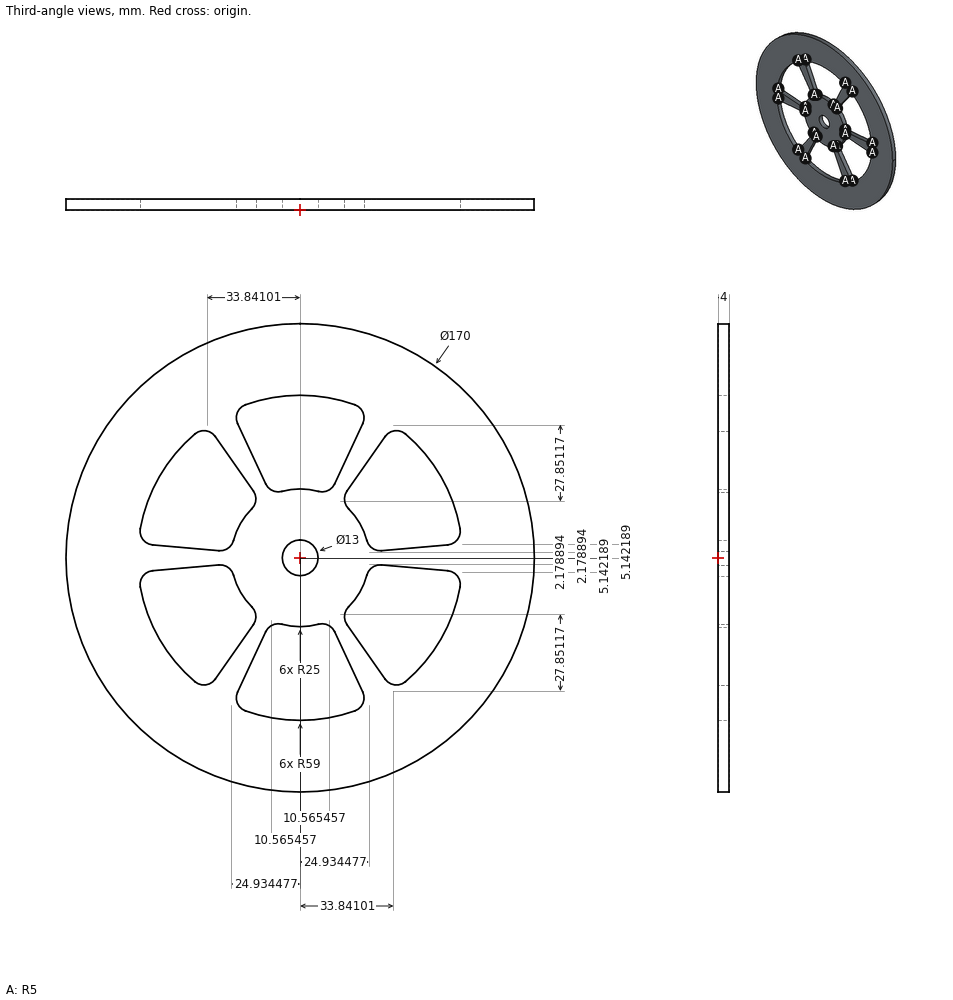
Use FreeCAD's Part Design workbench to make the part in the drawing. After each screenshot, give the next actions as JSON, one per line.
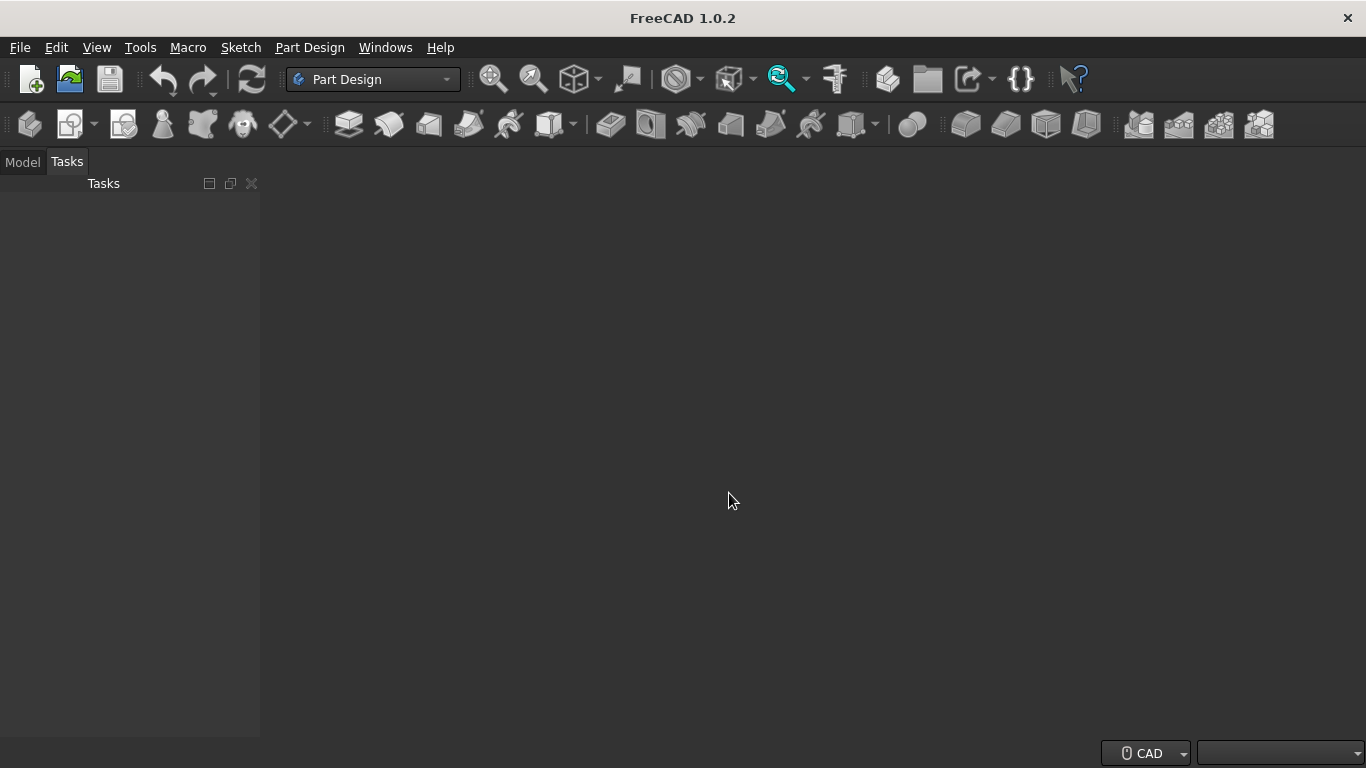
{"action": "left_click", "coordinate": [30, 80]}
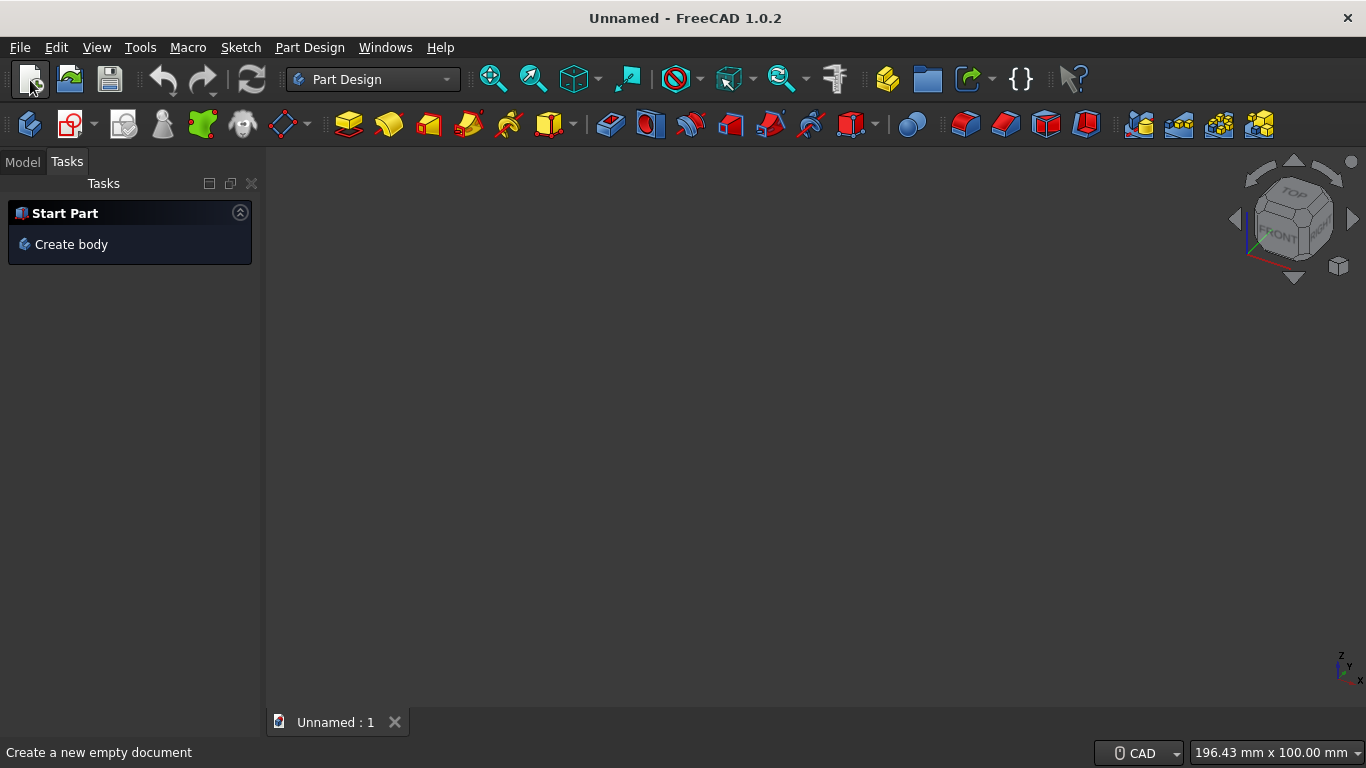
{"action": "left_click", "coordinate": [70, 124]}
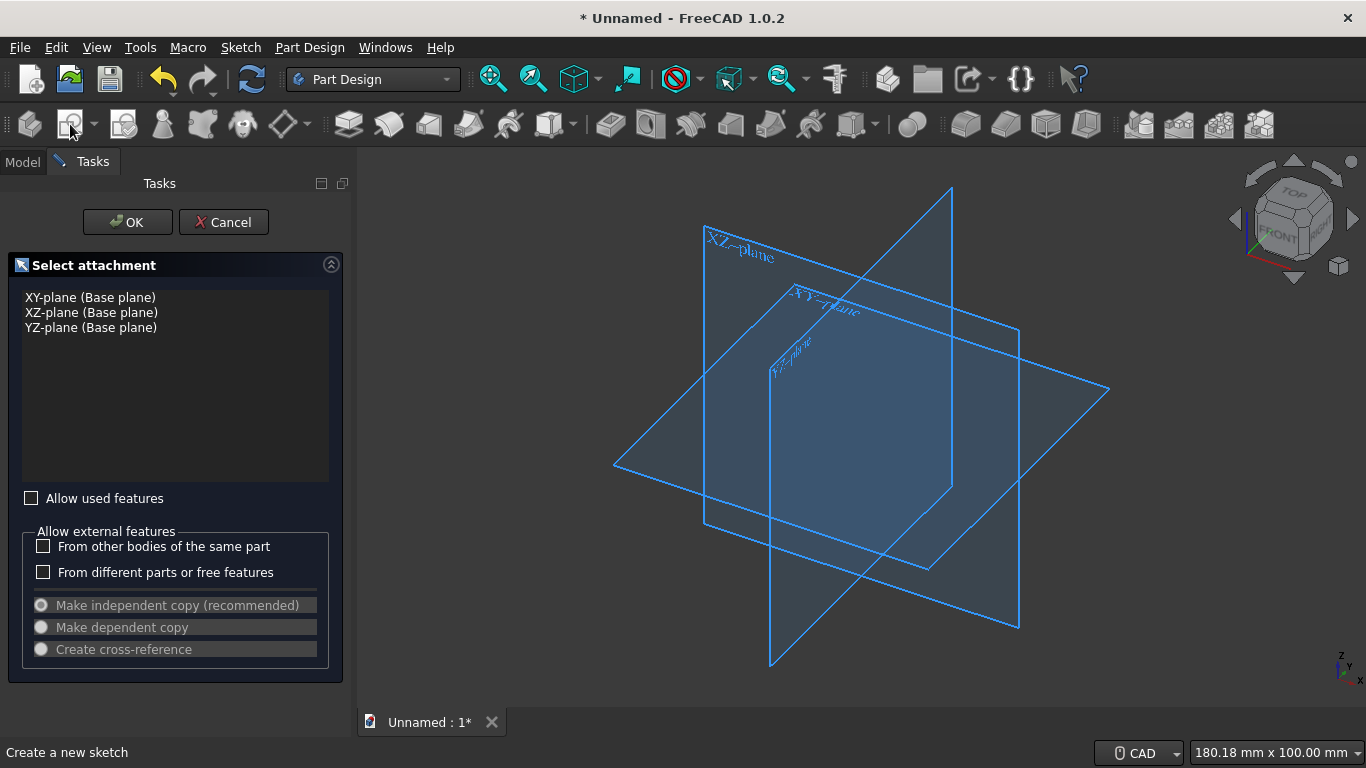
{"action": "left_click", "coordinate": [82, 312]}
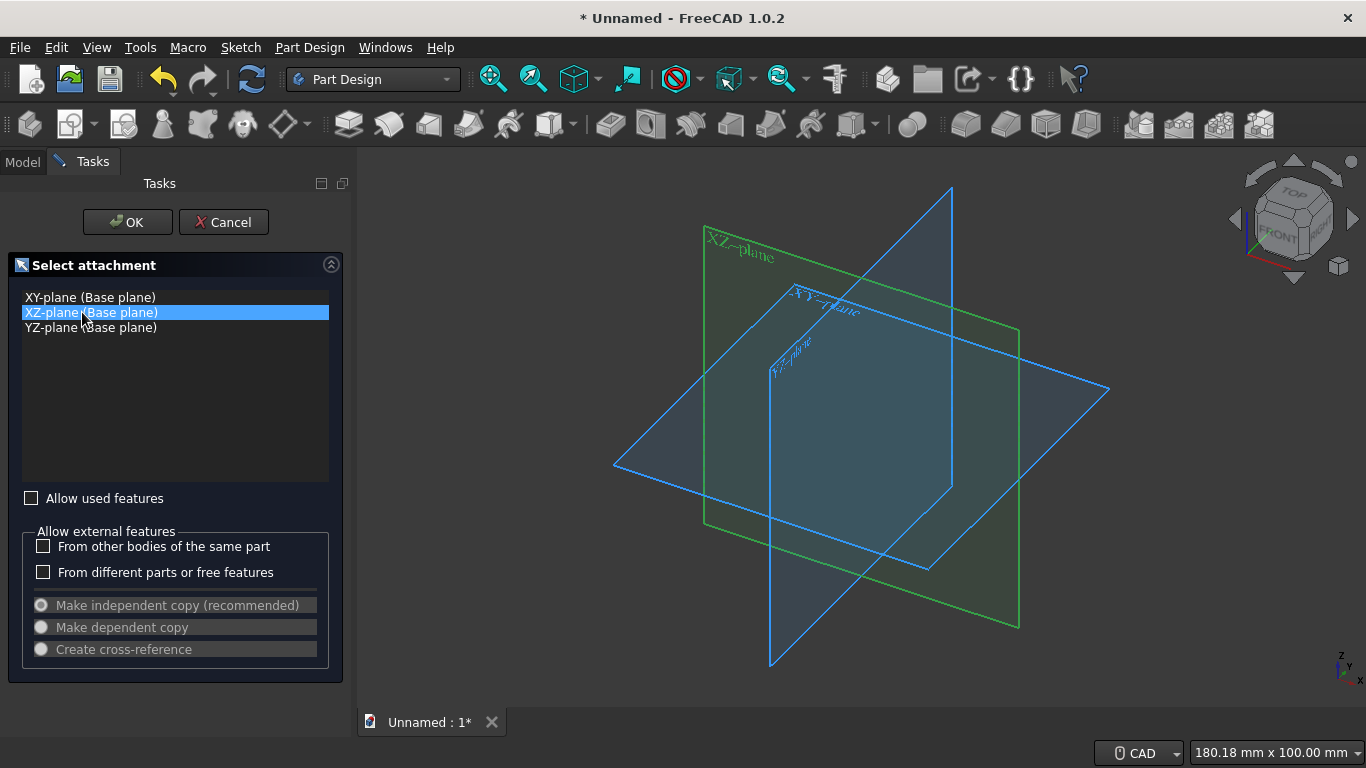
{"action": "left_click", "coordinate": [128, 222]}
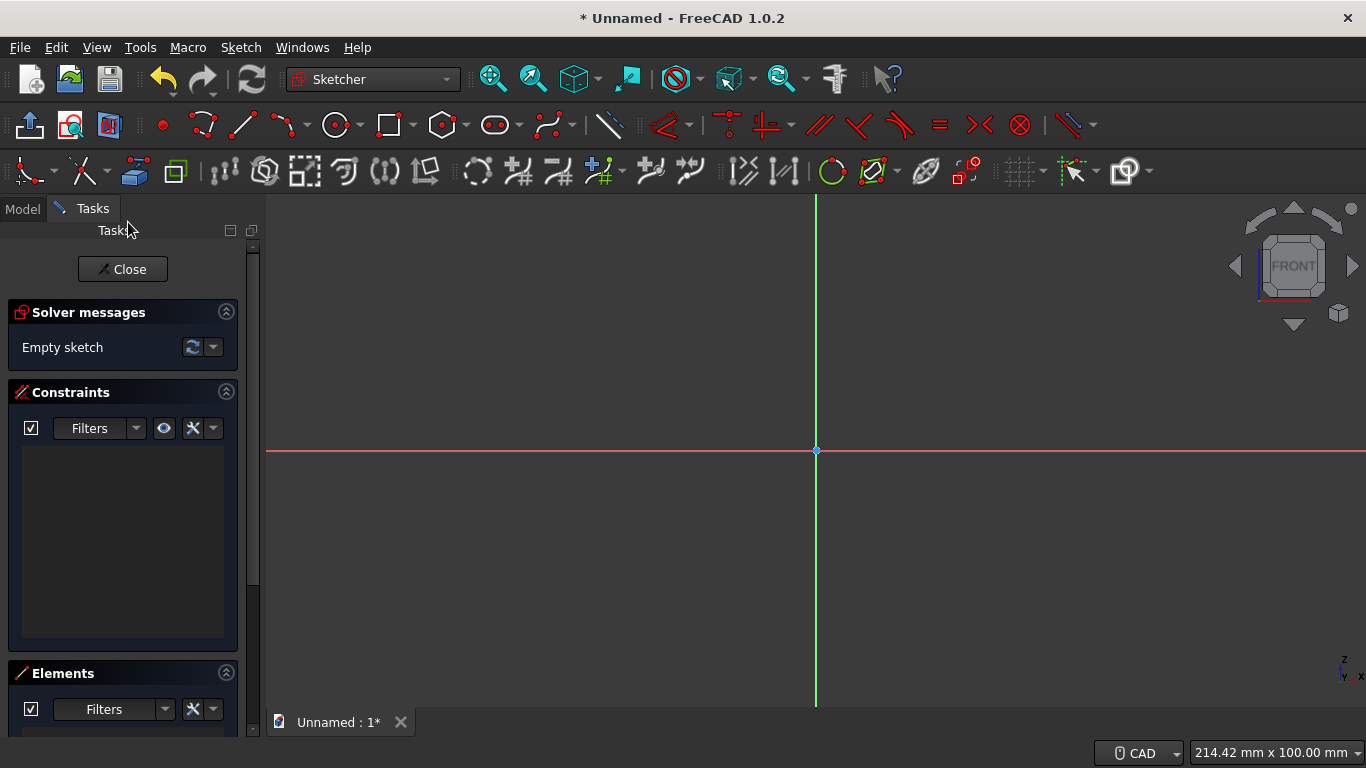
{"action": "scroll", "coordinate": [708, 450], "scroll_direction": "down", "scroll_amount": 5}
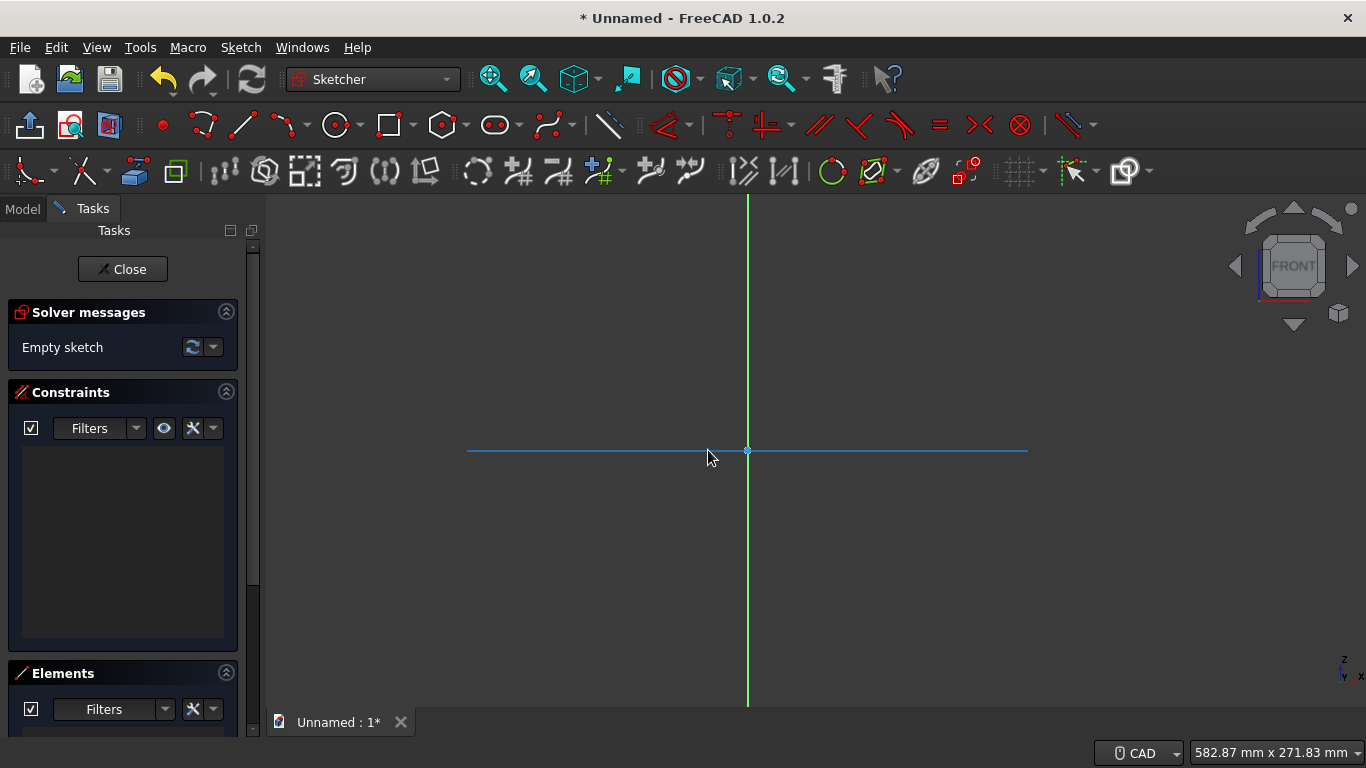
{"action": "left_click", "coordinate": [336, 126]}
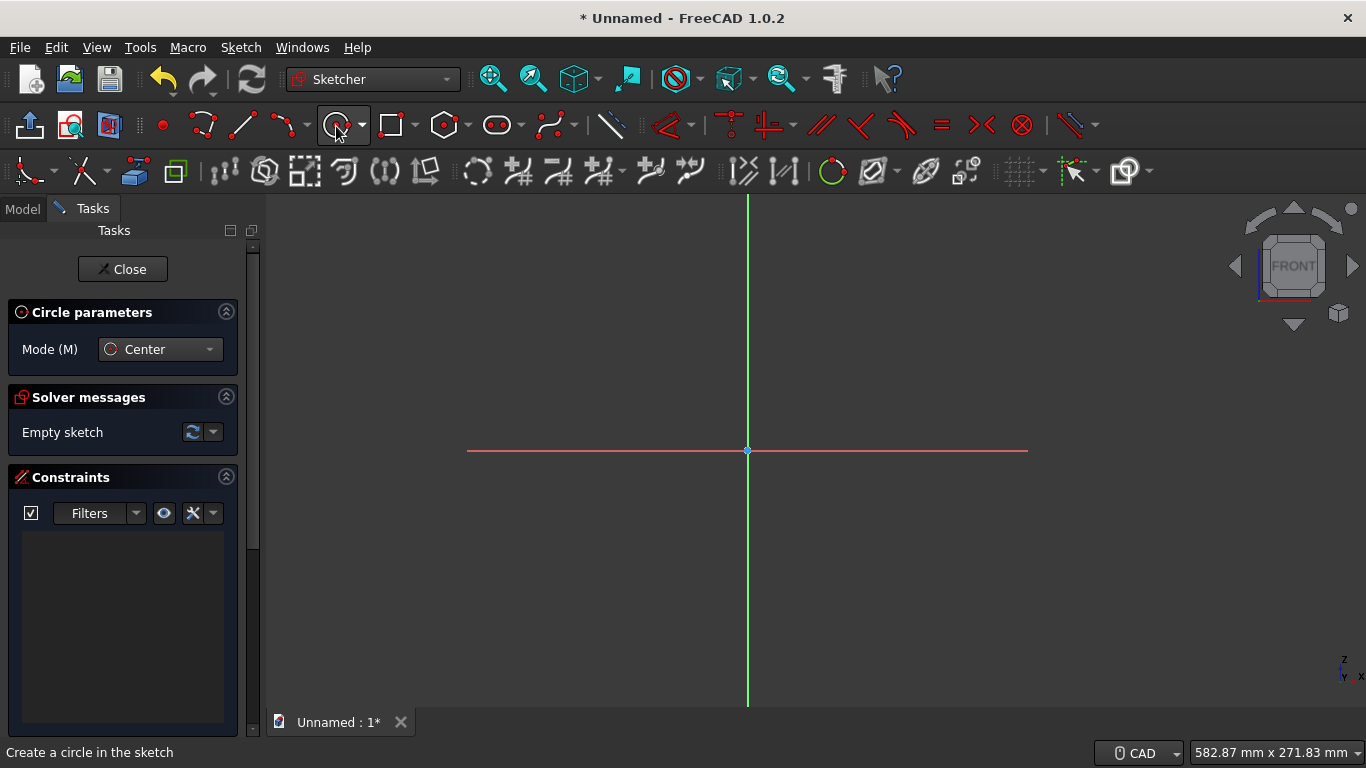
{"action": "left_click", "coordinate": [748, 450]}
{"action": "mouse_move", "coordinate": [861, 337]}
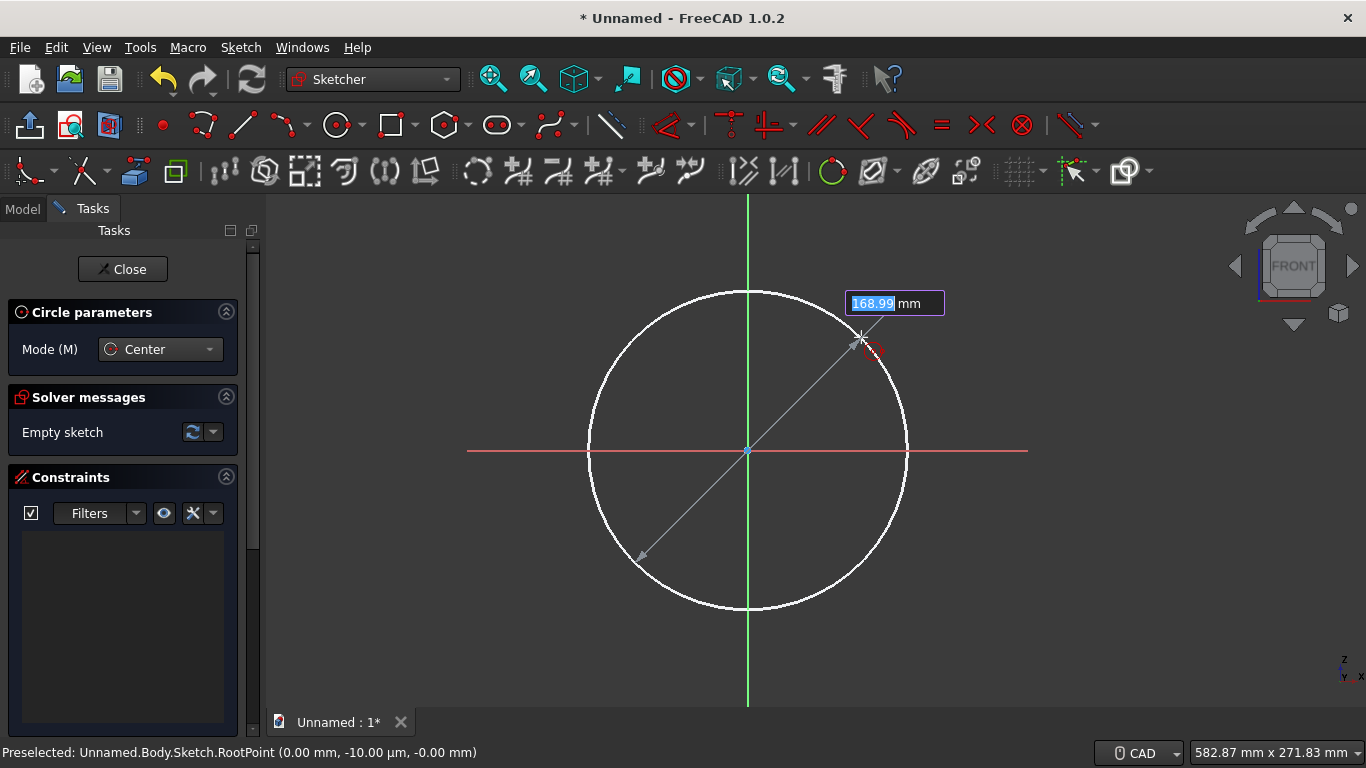
{"action": "type", "text": "170"}
{"action": "key", "text": "Return"}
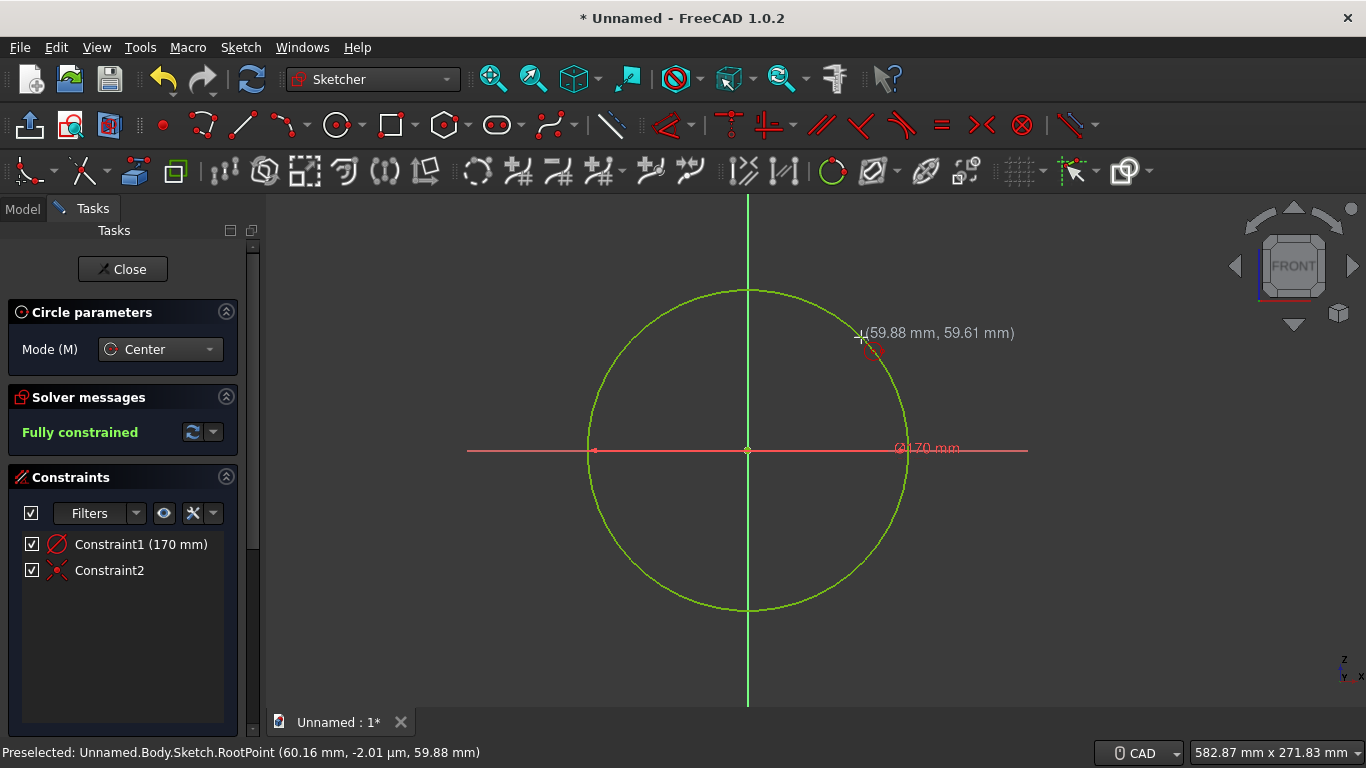
{"action": "scroll", "coordinate": [748, 450], "scroll_direction": "up", "scroll_amount": 4}